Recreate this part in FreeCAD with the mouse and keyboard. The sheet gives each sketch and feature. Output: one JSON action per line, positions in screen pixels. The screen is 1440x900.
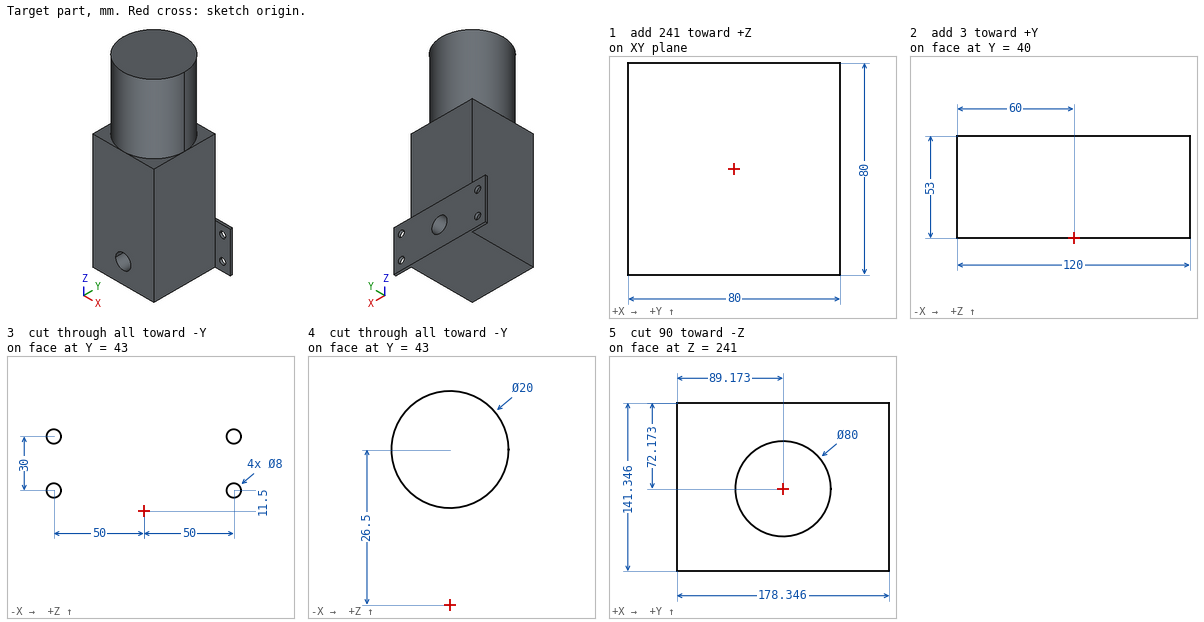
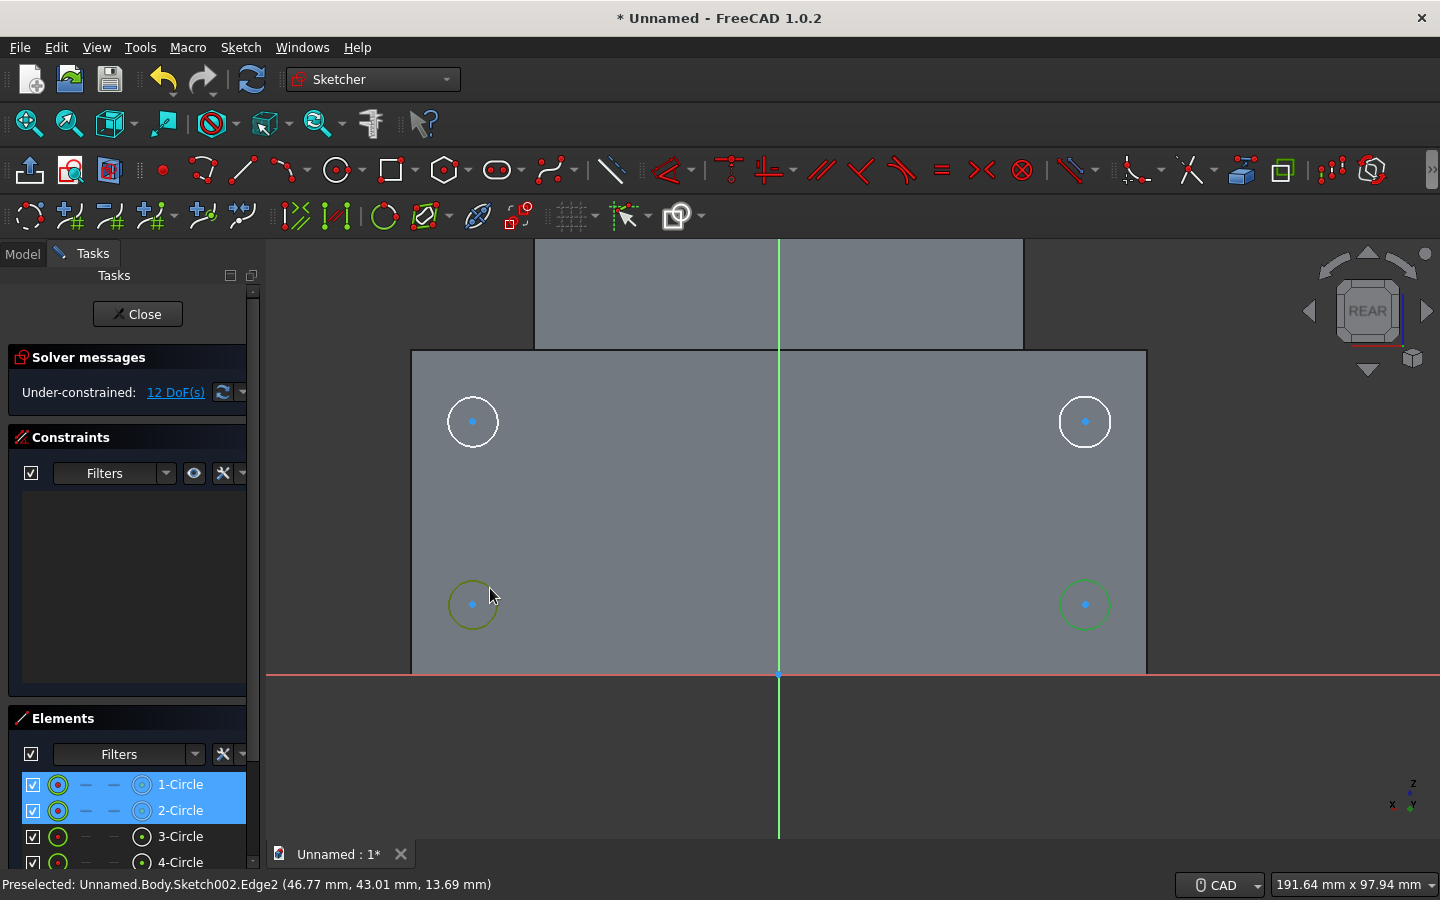
{"action": "left_click", "coordinate": [490, 404]}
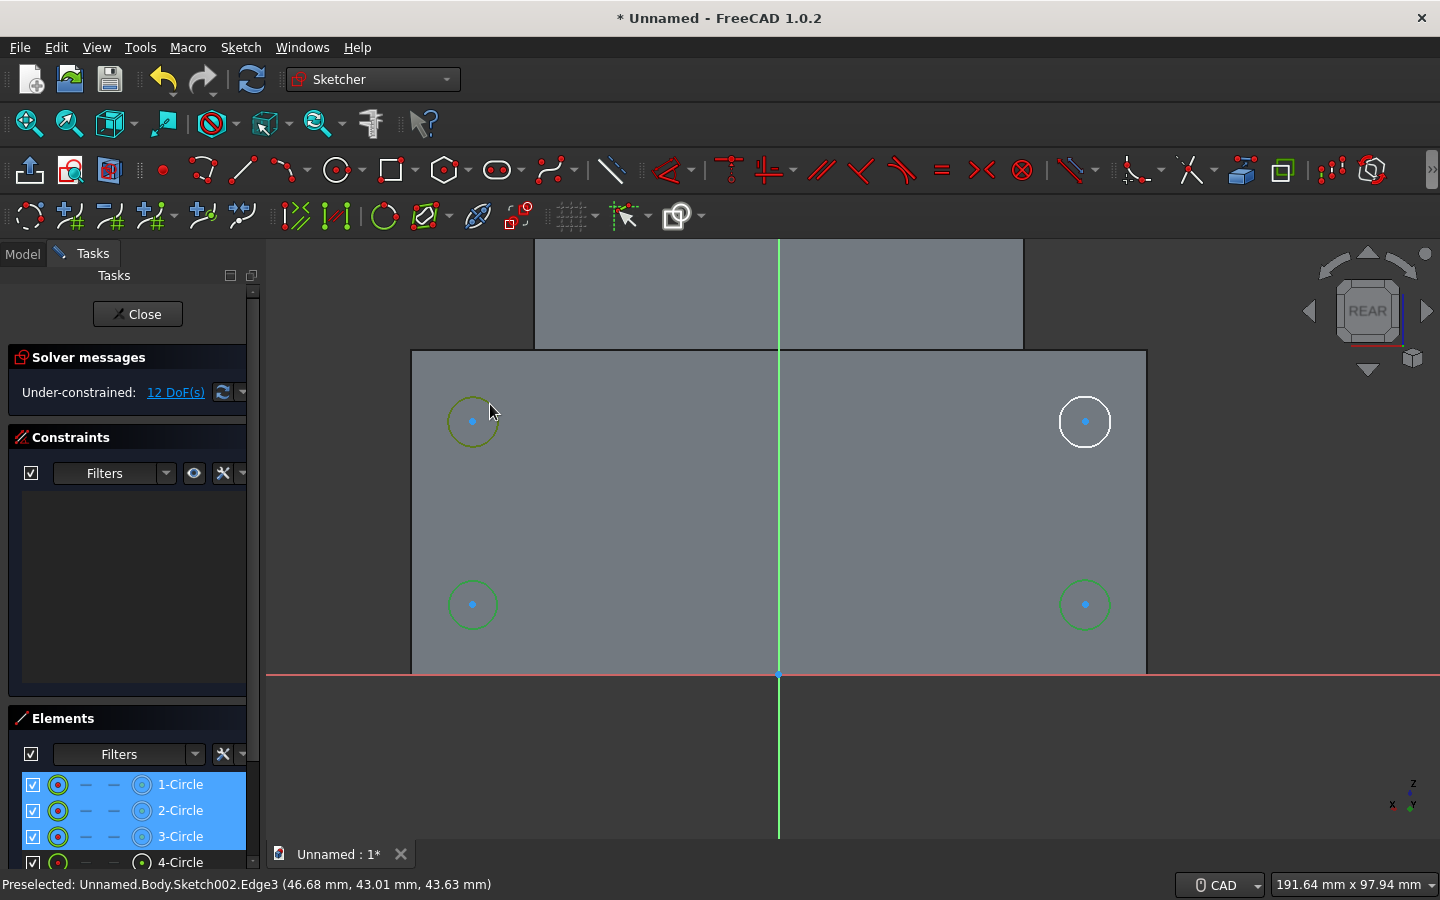
{"action": "left_click", "coordinate": [1103, 404]}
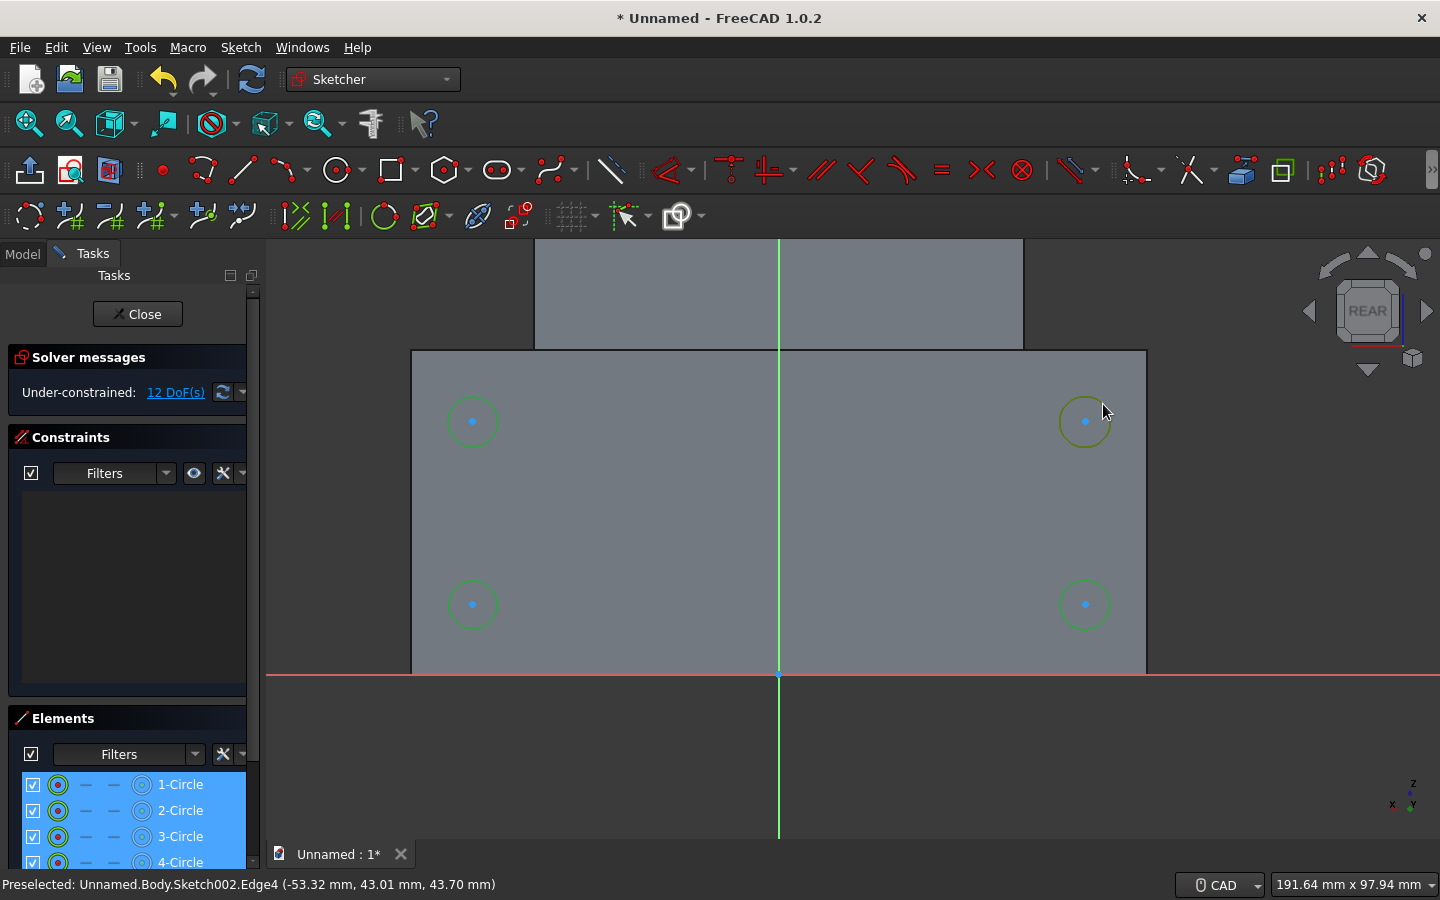
{"action": "key", "text": "e"}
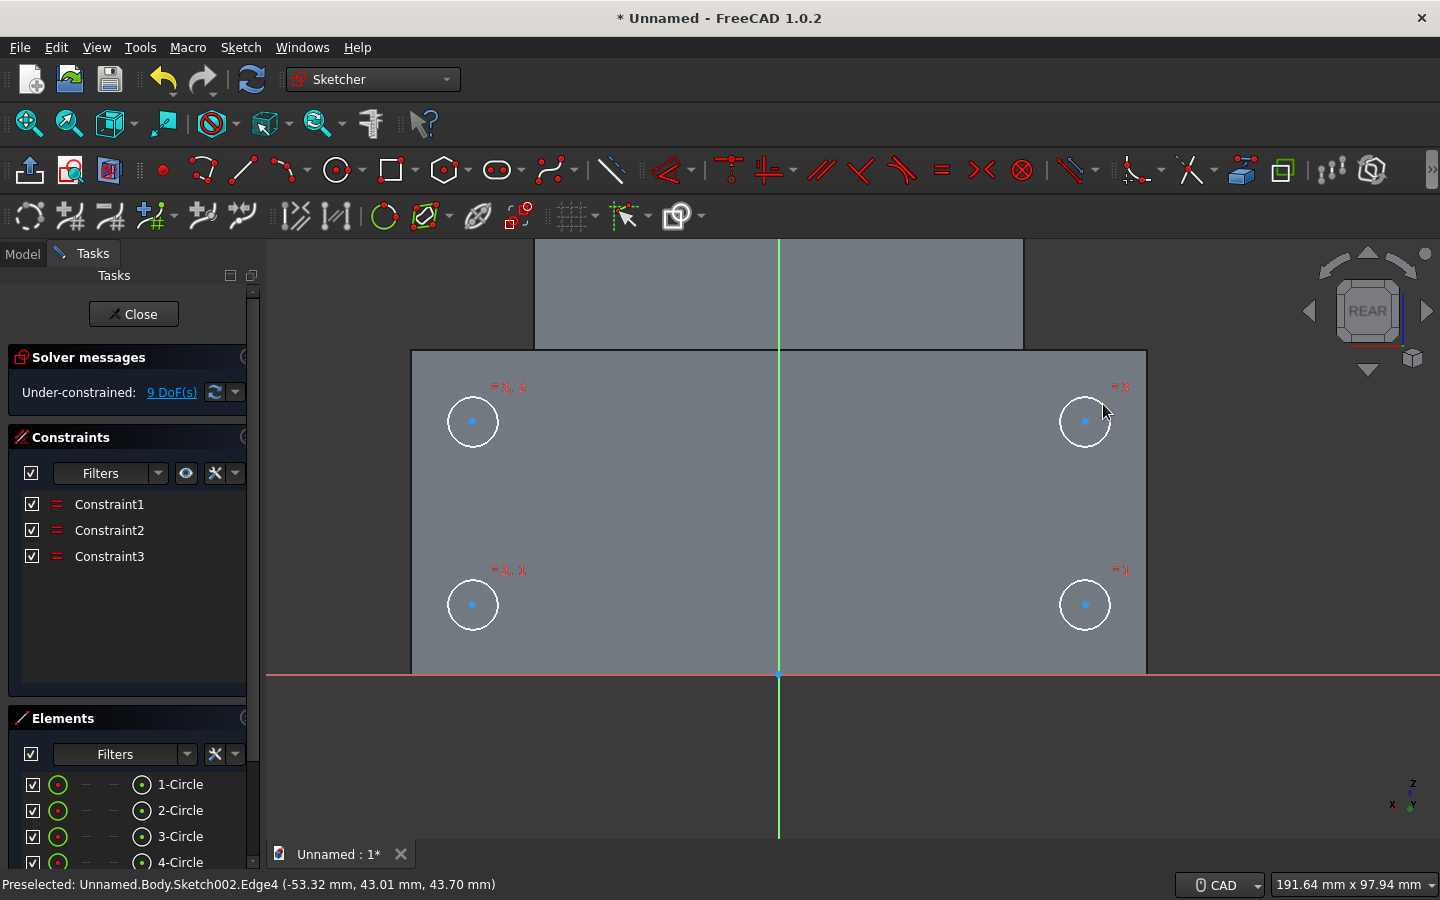
{"action": "left_click", "coordinate": [1085, 605]}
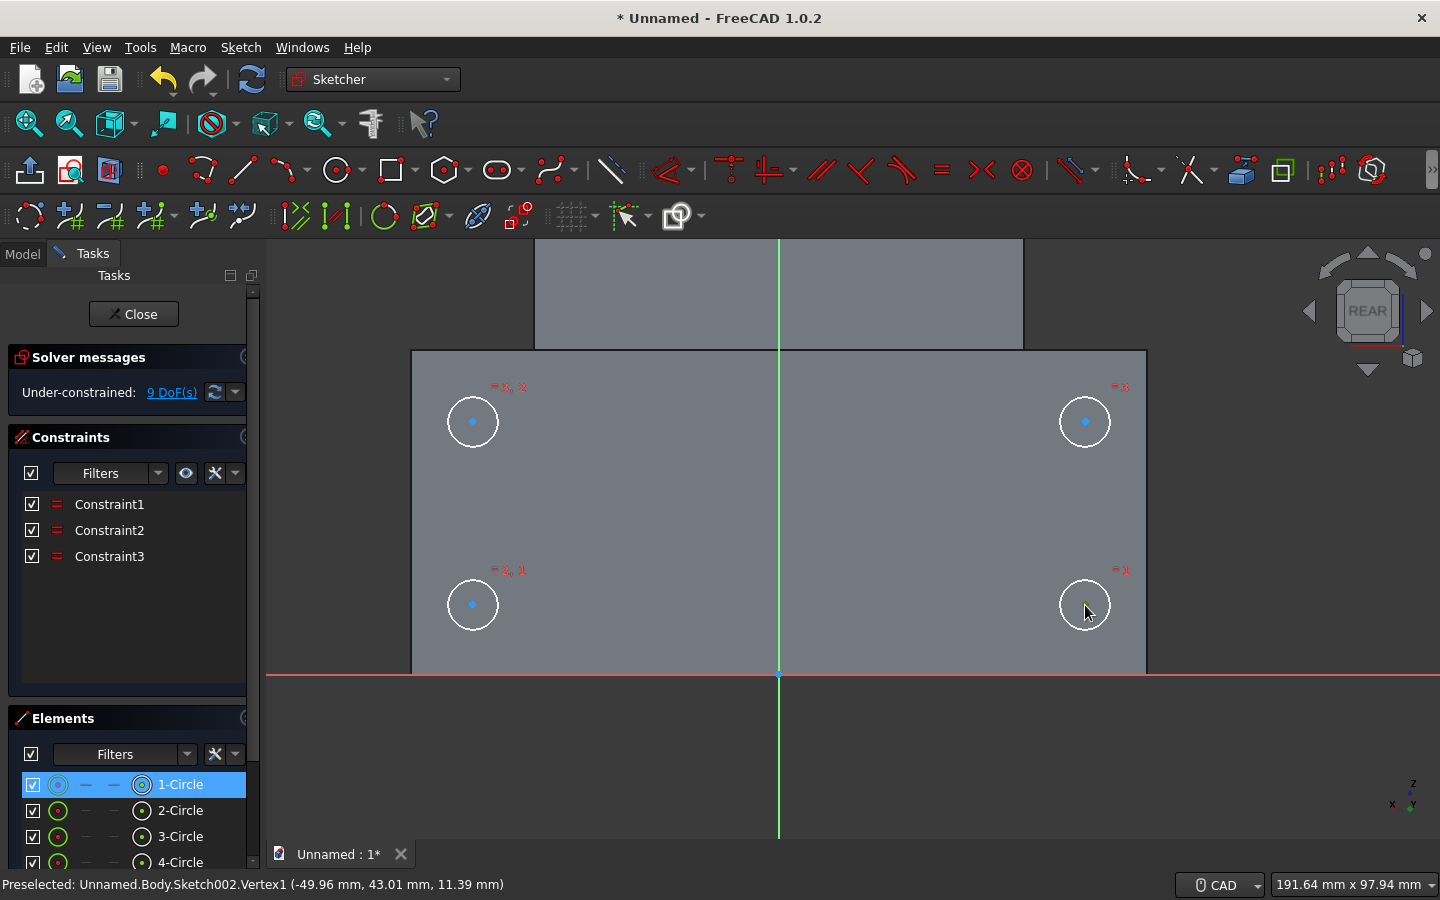
{"action": "left_click", "coordinate": [473, 605]}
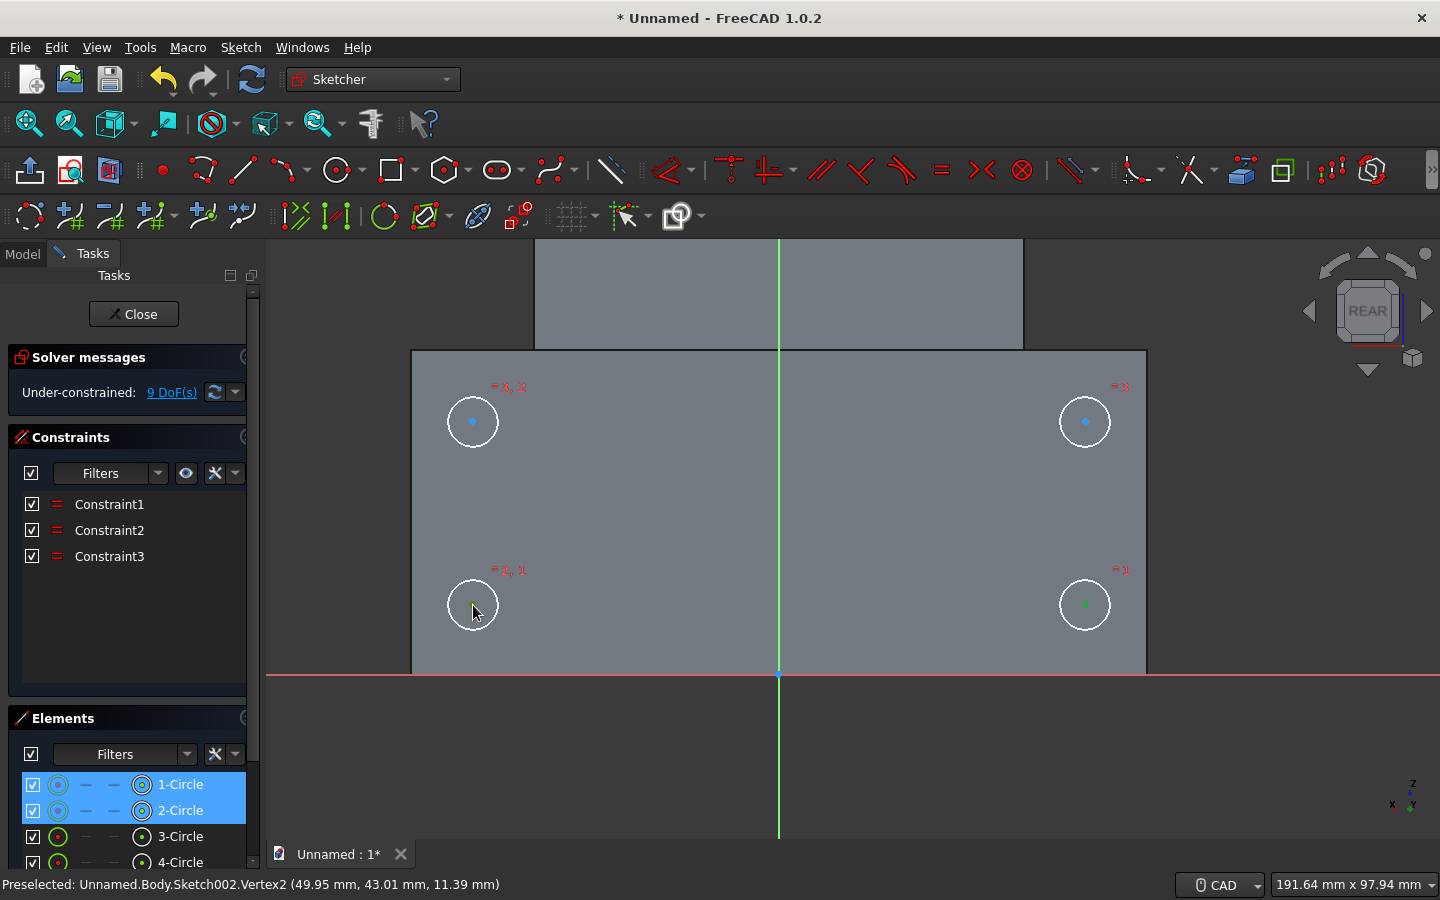
{"action": "key", "text": "h"}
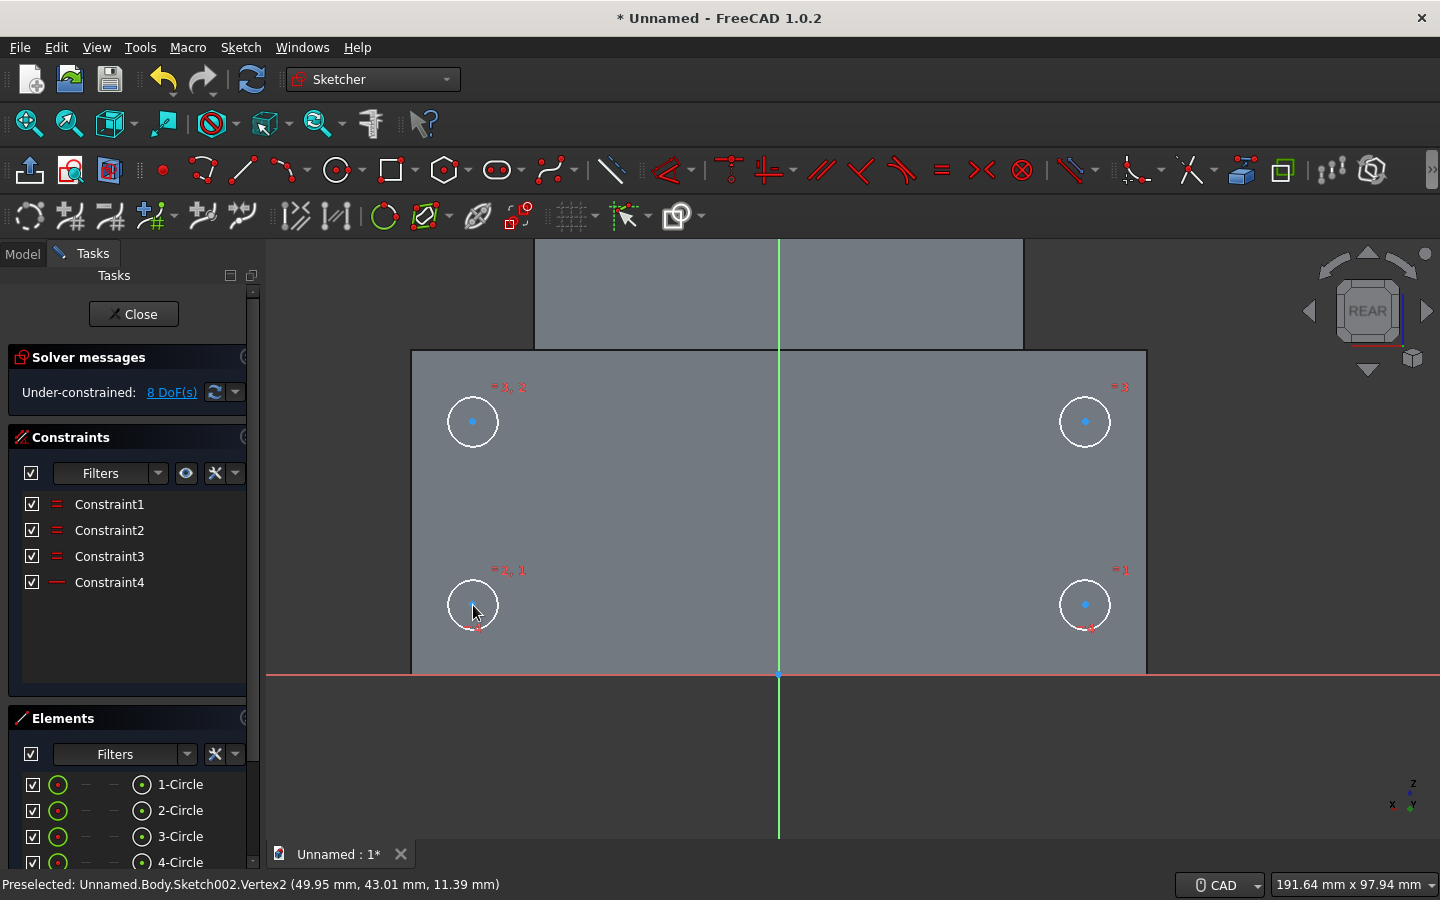
{"action": "left_click", "coordinate": [473, 605]}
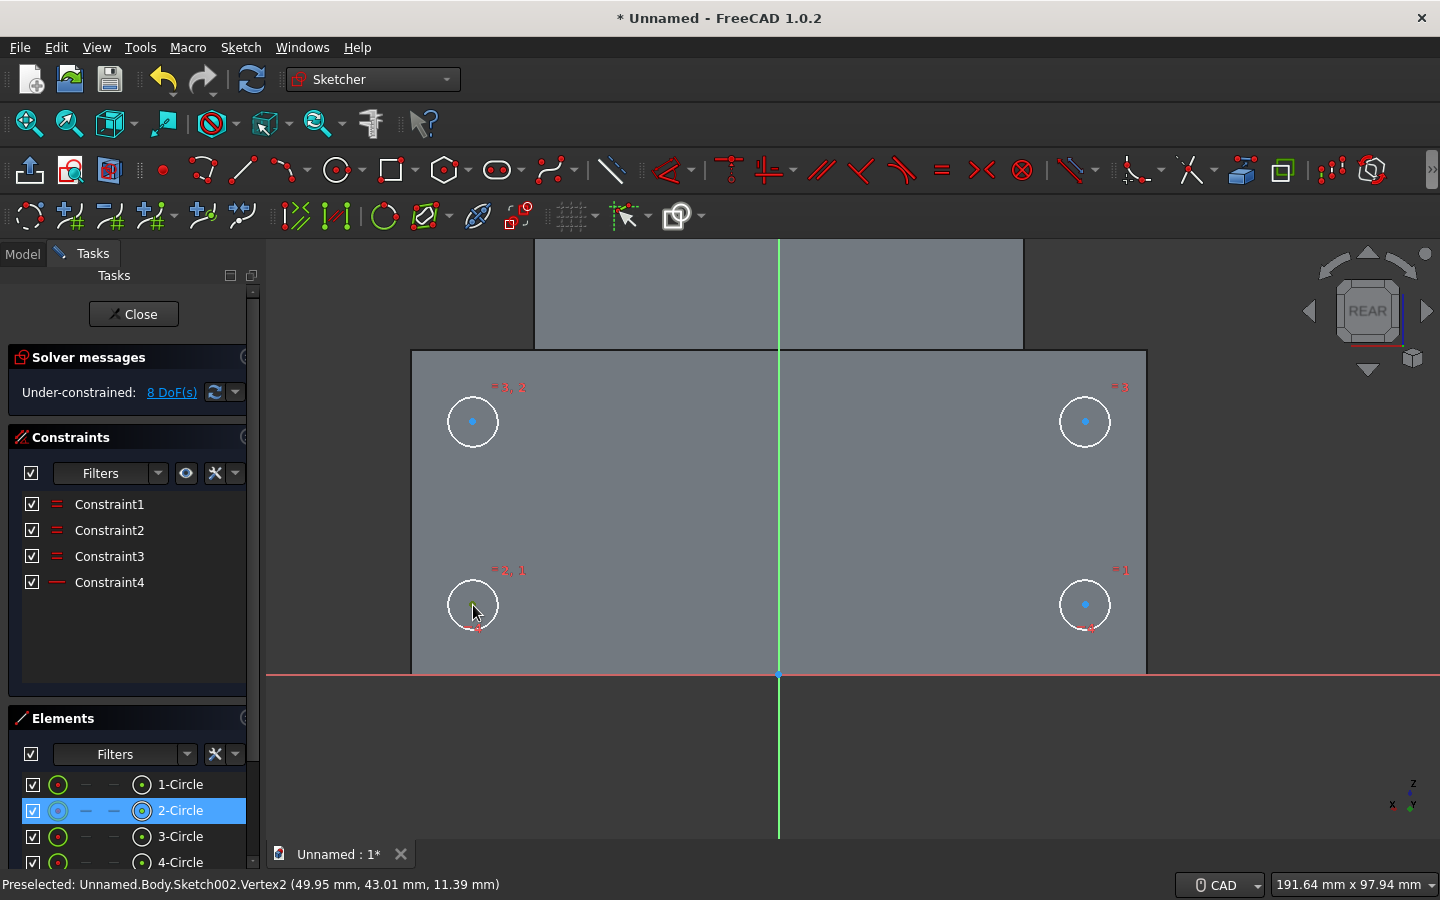
{"action": "left_click", "coordinate": [473, 422]}